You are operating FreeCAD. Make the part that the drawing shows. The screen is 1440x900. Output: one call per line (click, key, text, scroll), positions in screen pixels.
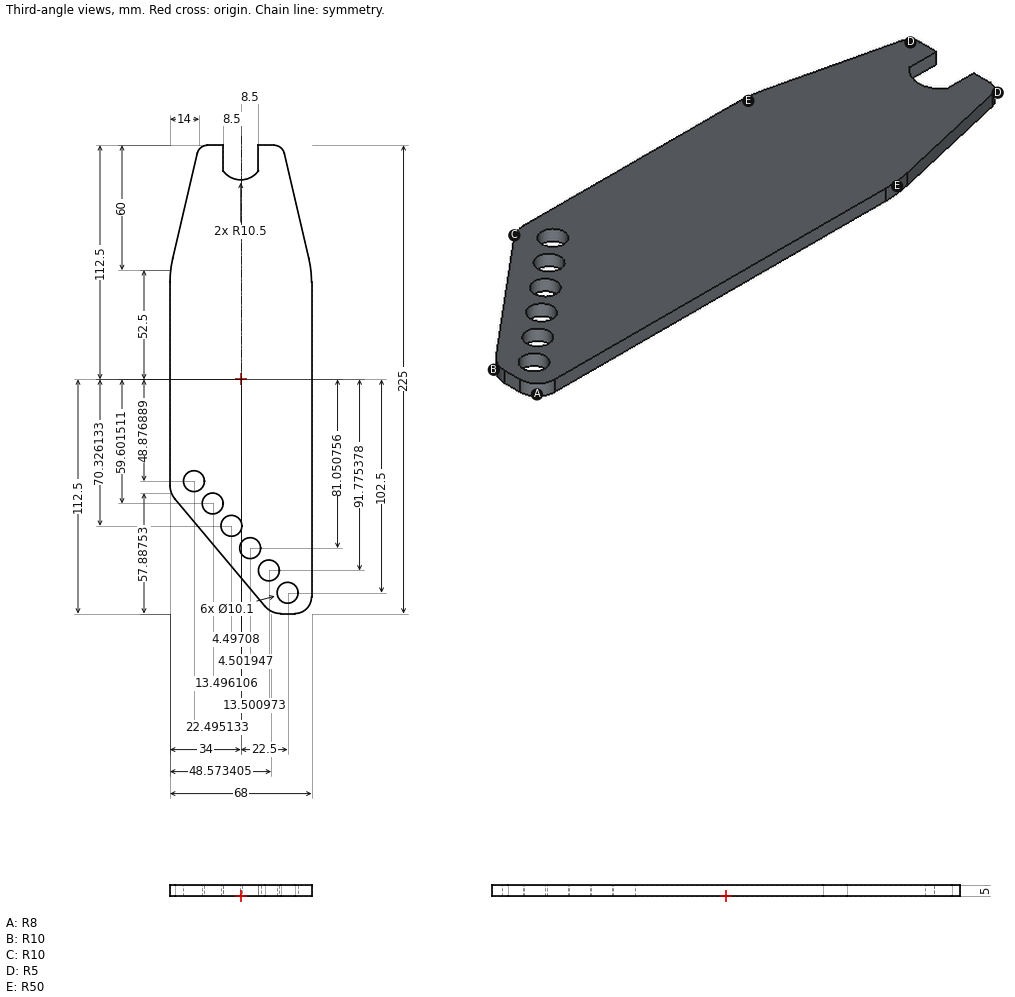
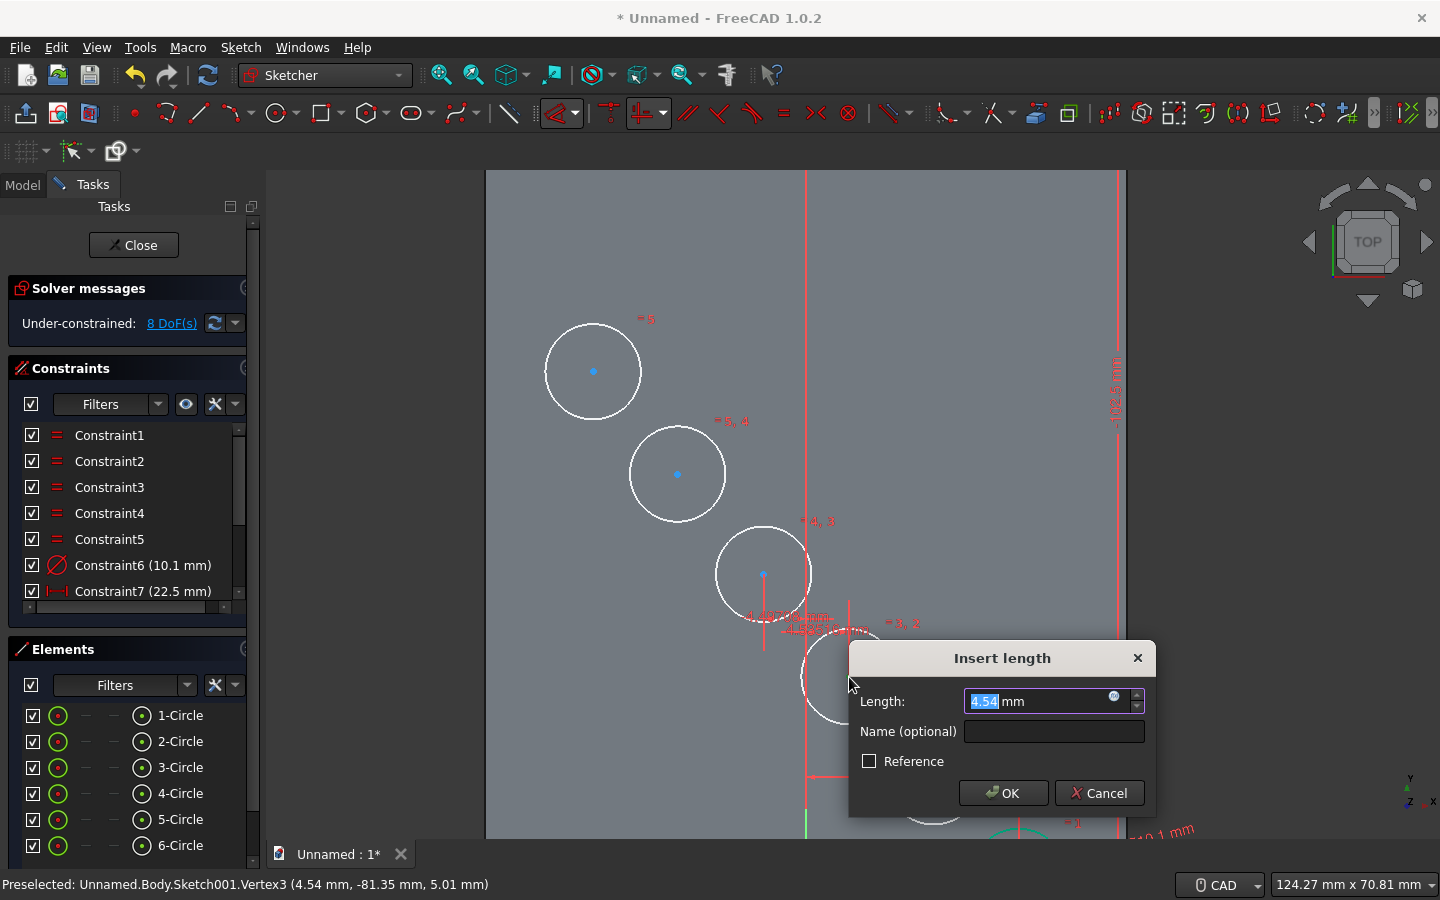
text(4.501947)
key(Return)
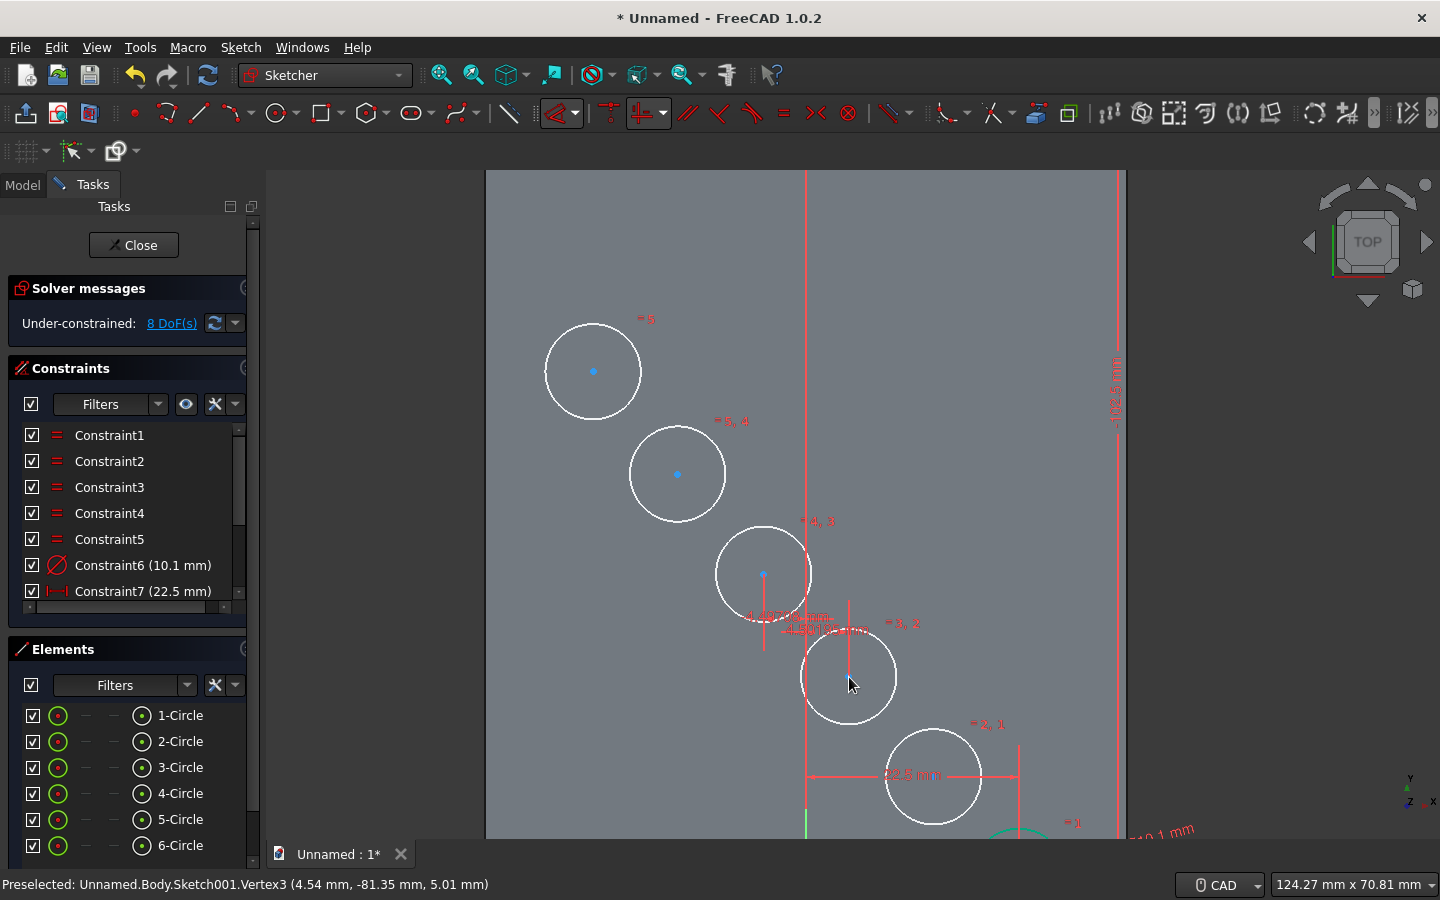
click(934, 777)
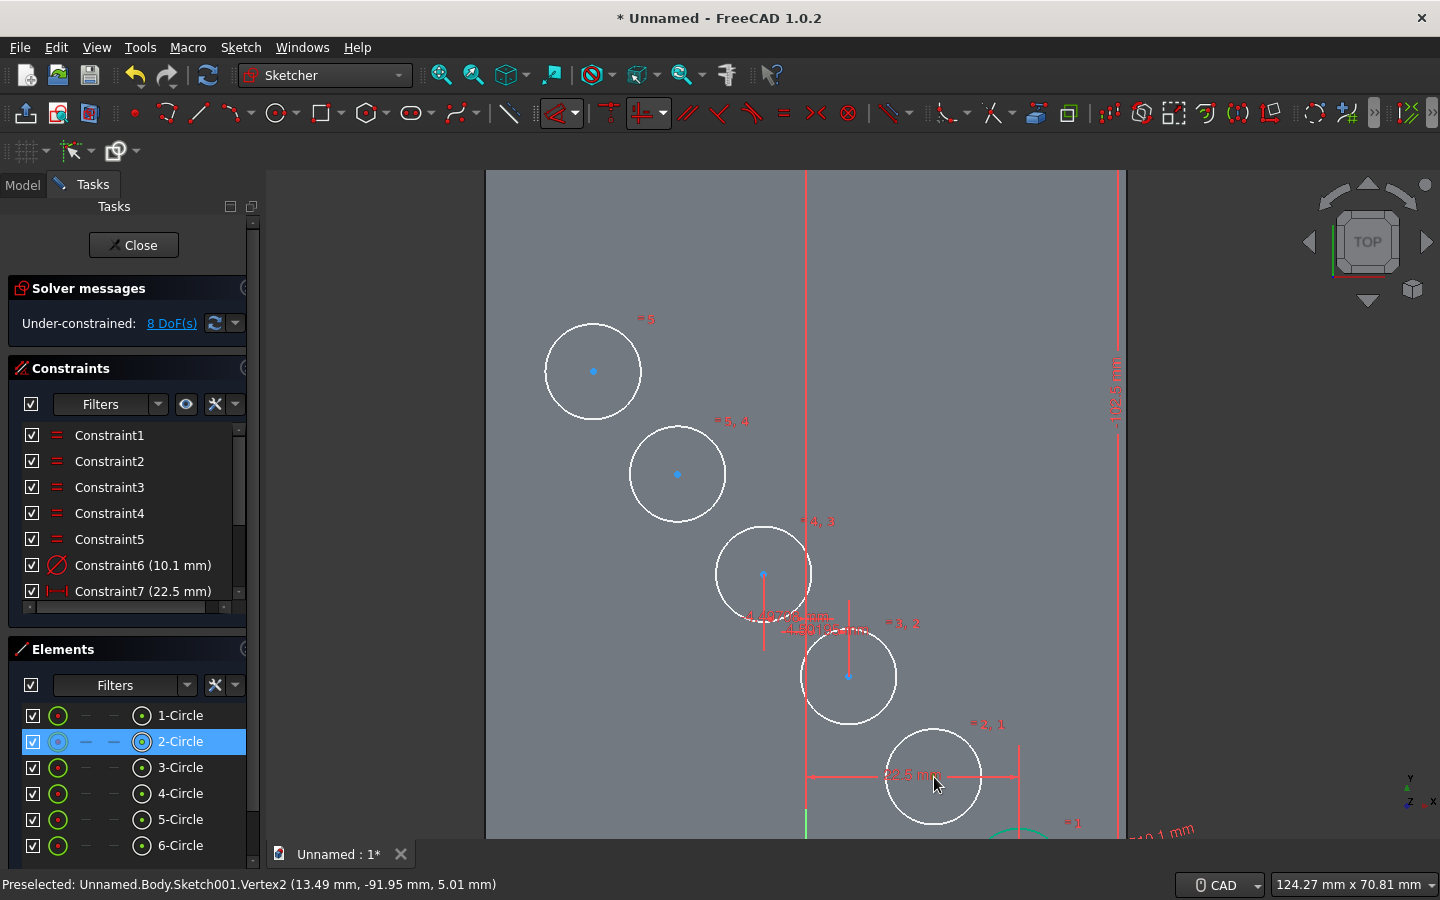
key(l)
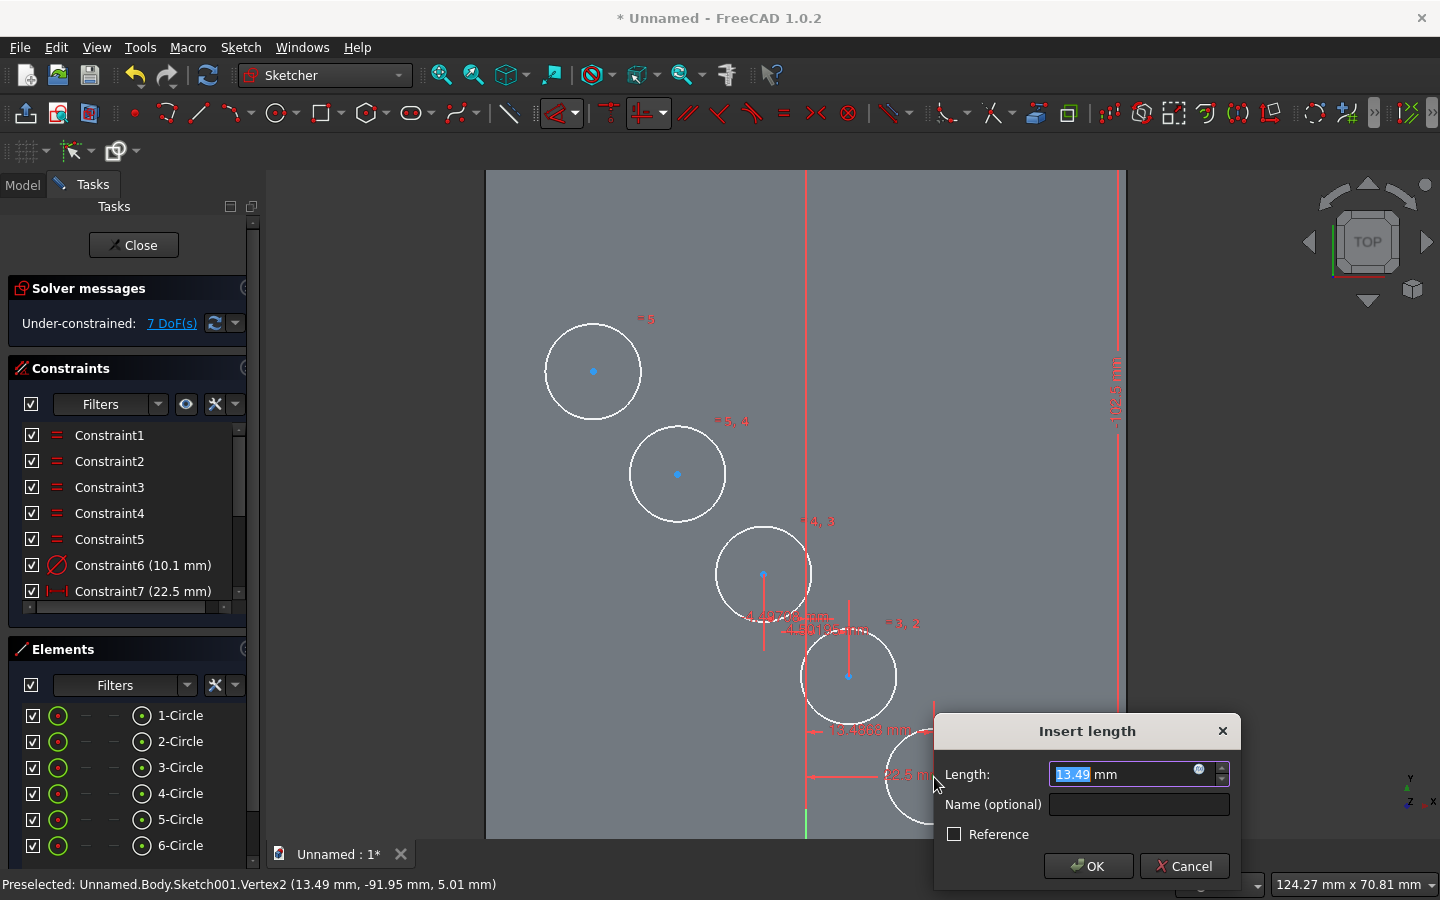
text(13.500973)
key(Return)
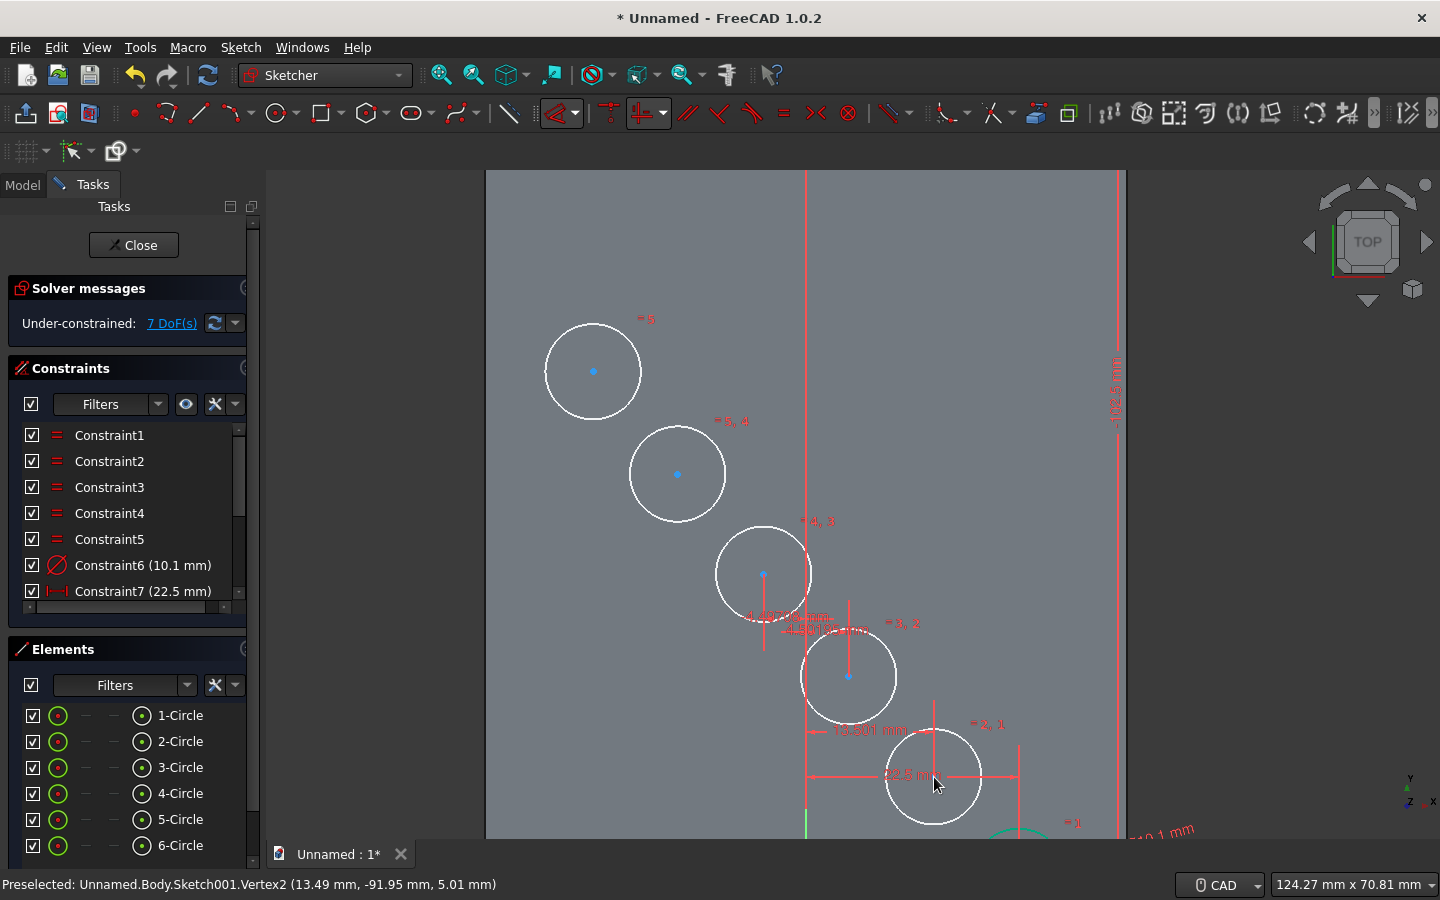
click(934, 777)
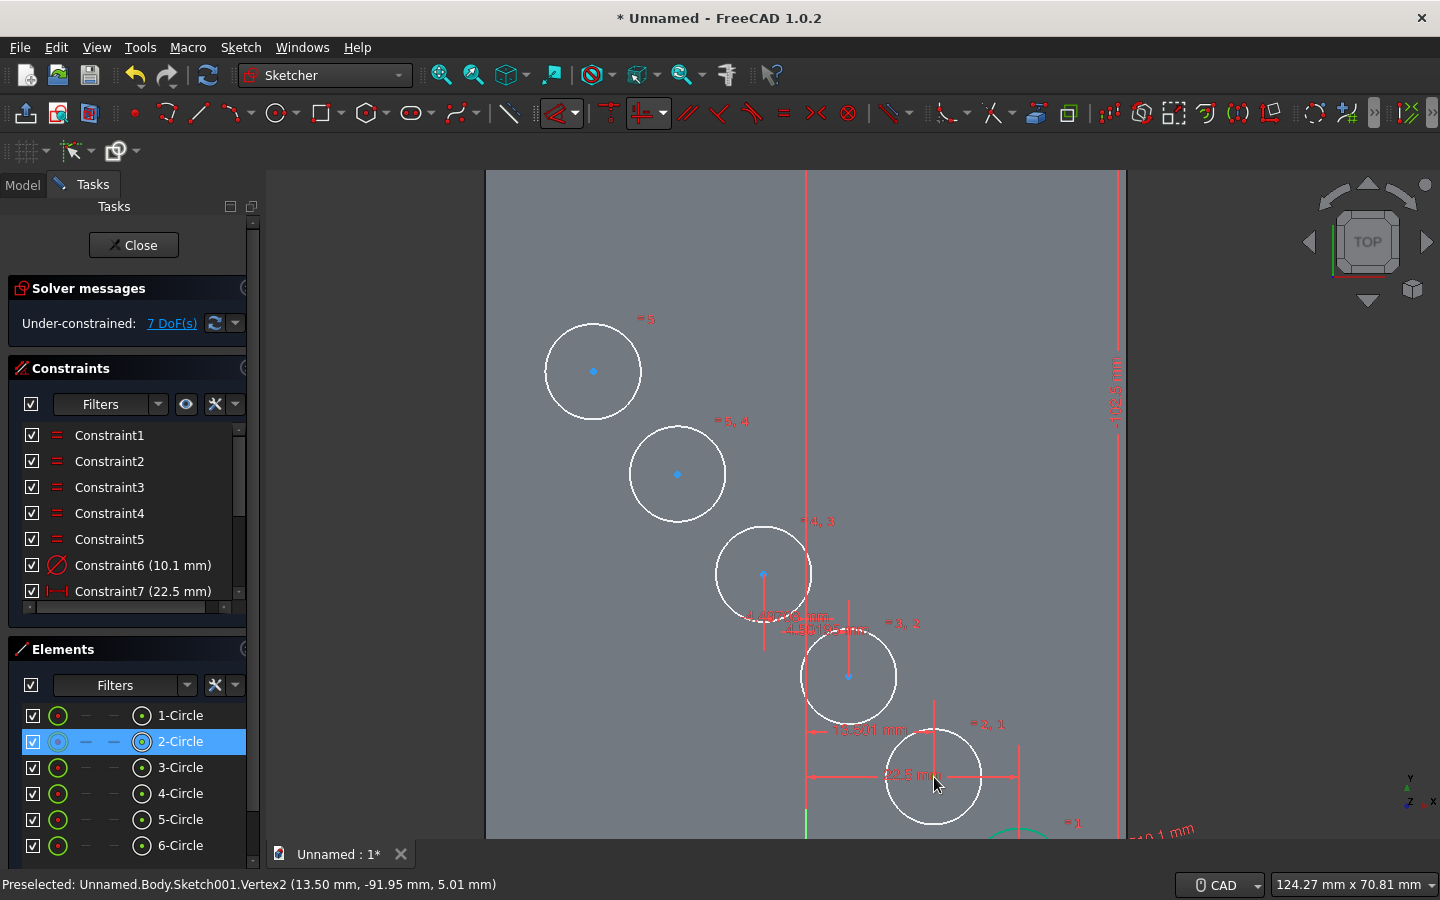
key(i)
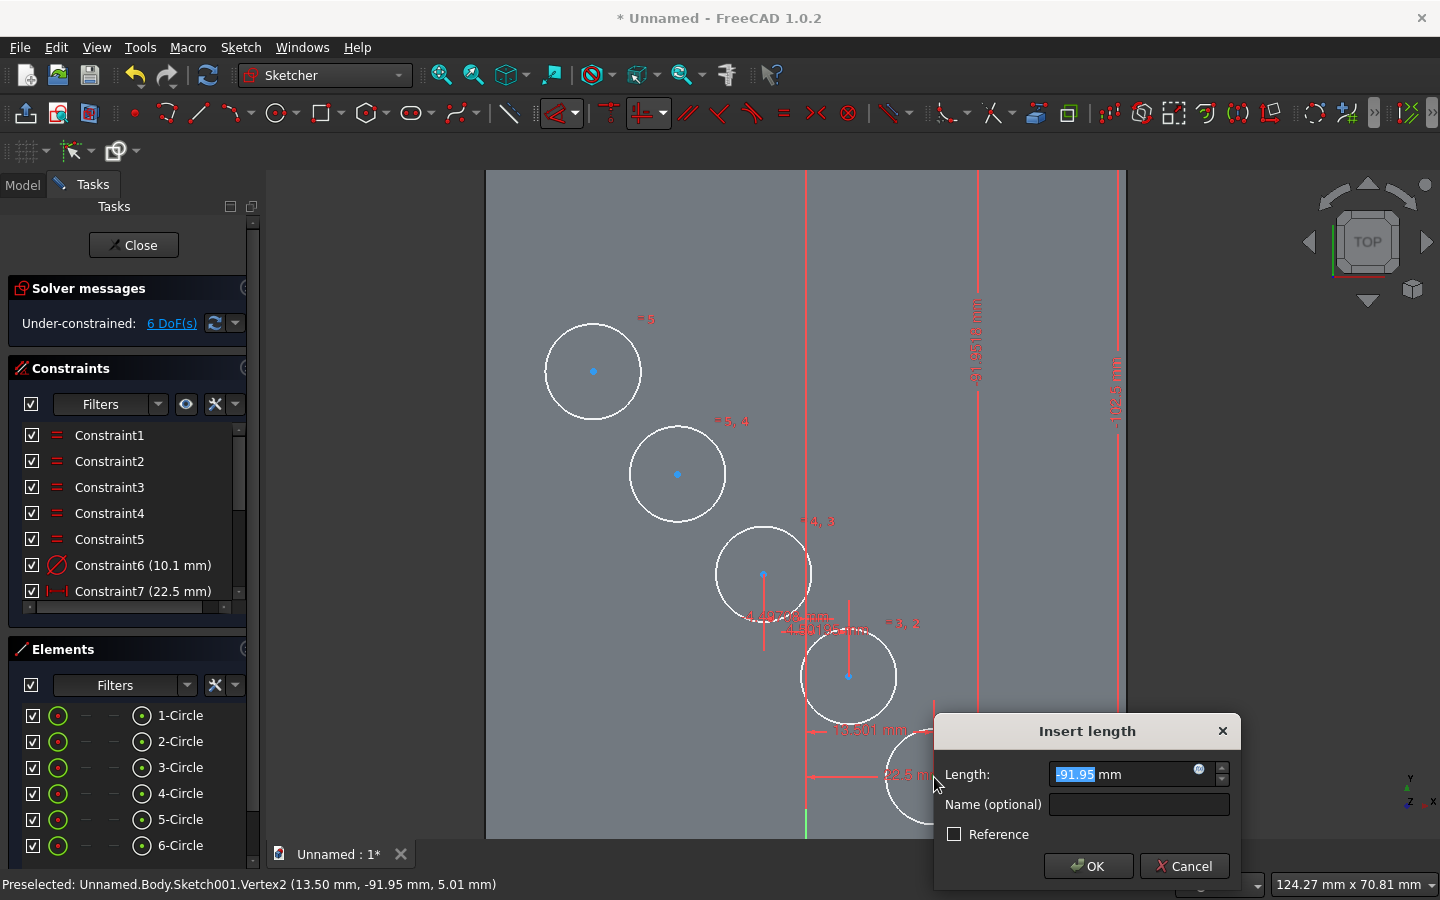
text(-91.775378)
key(Return)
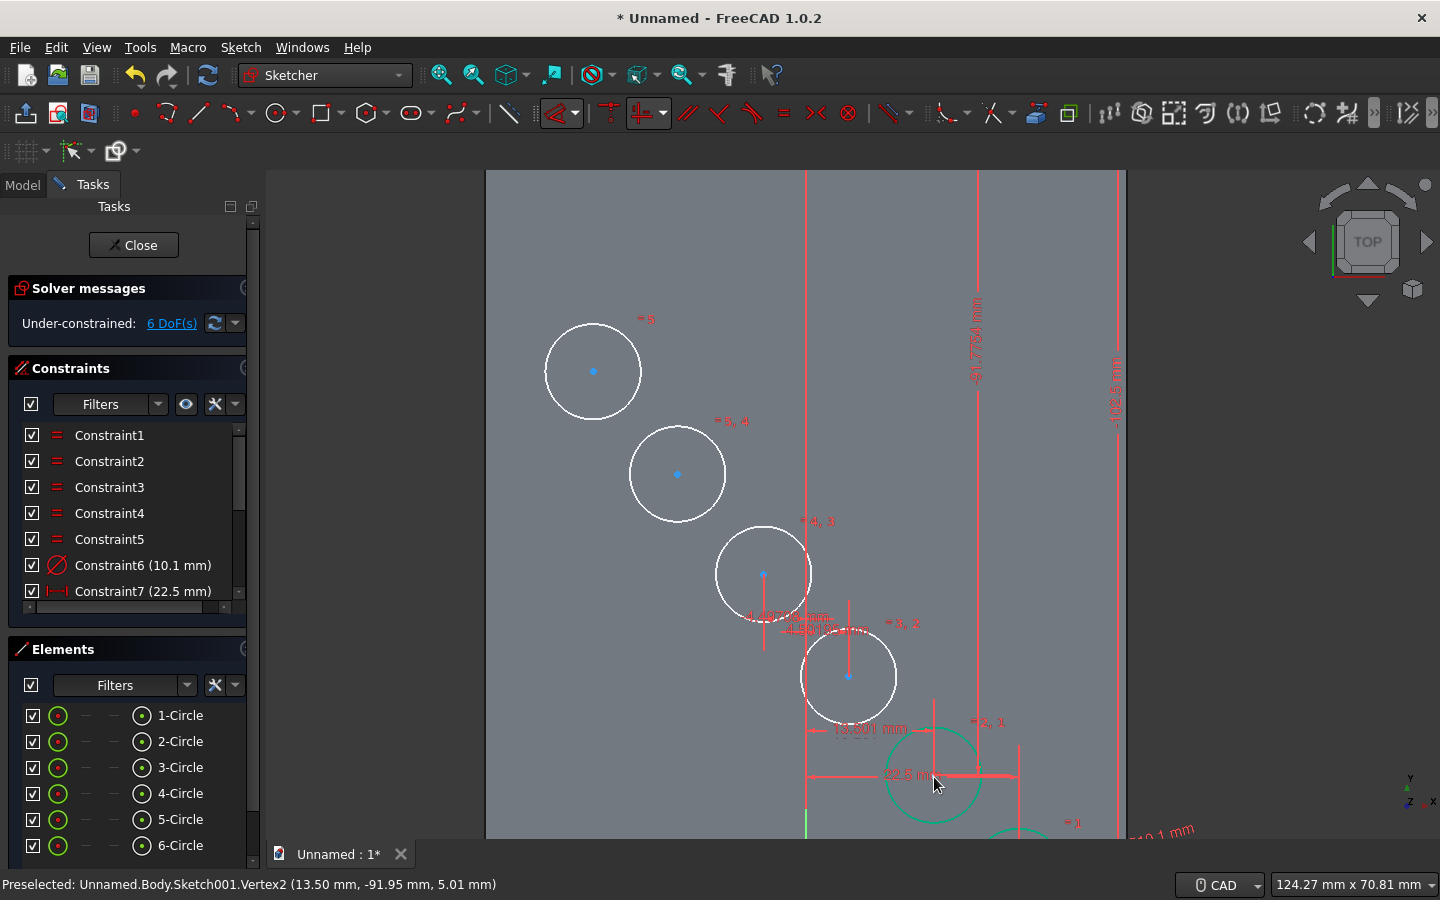
click(849, 677)